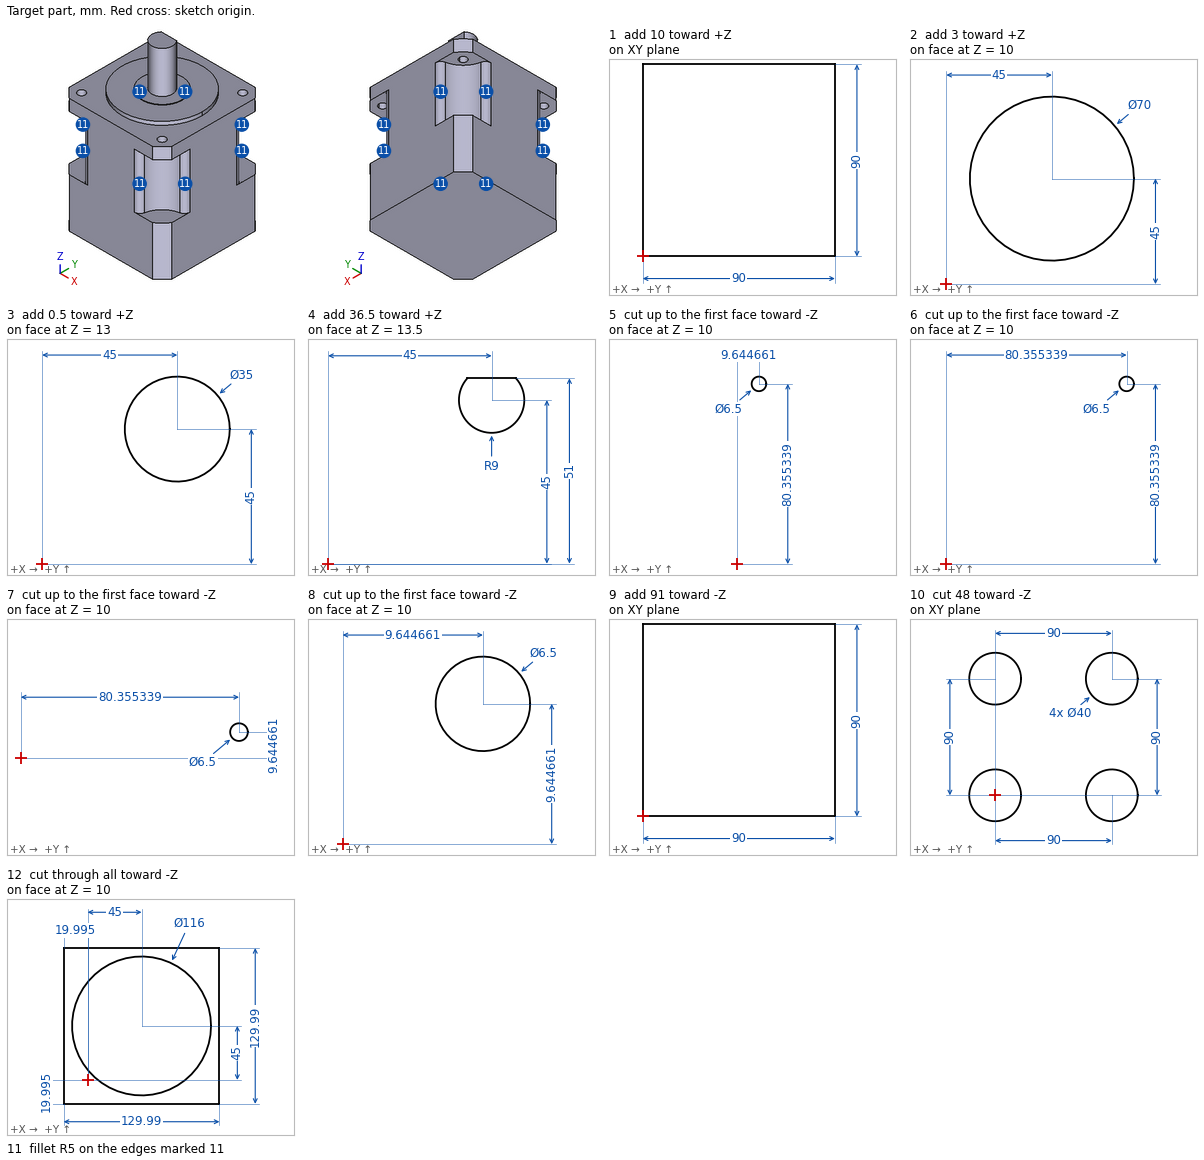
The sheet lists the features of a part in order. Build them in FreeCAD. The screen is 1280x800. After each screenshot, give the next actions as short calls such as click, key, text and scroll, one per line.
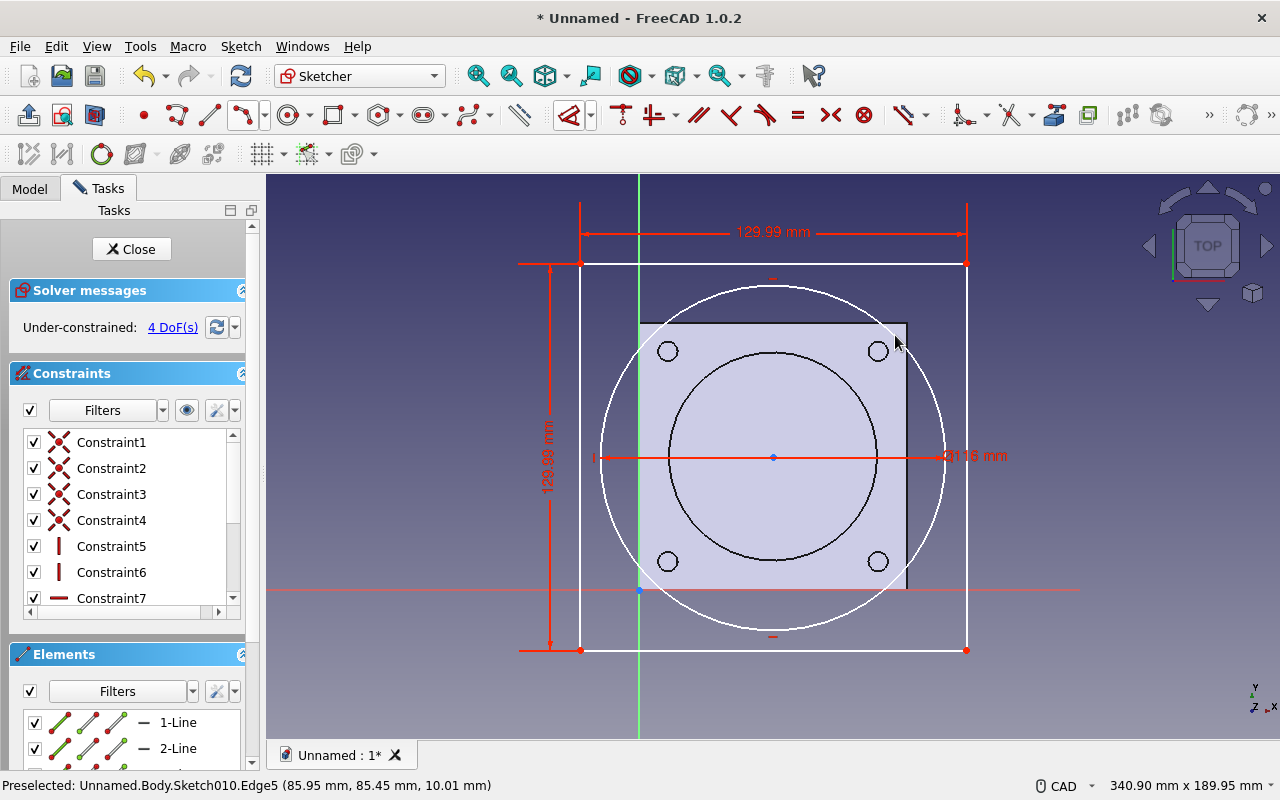
click(773, 458)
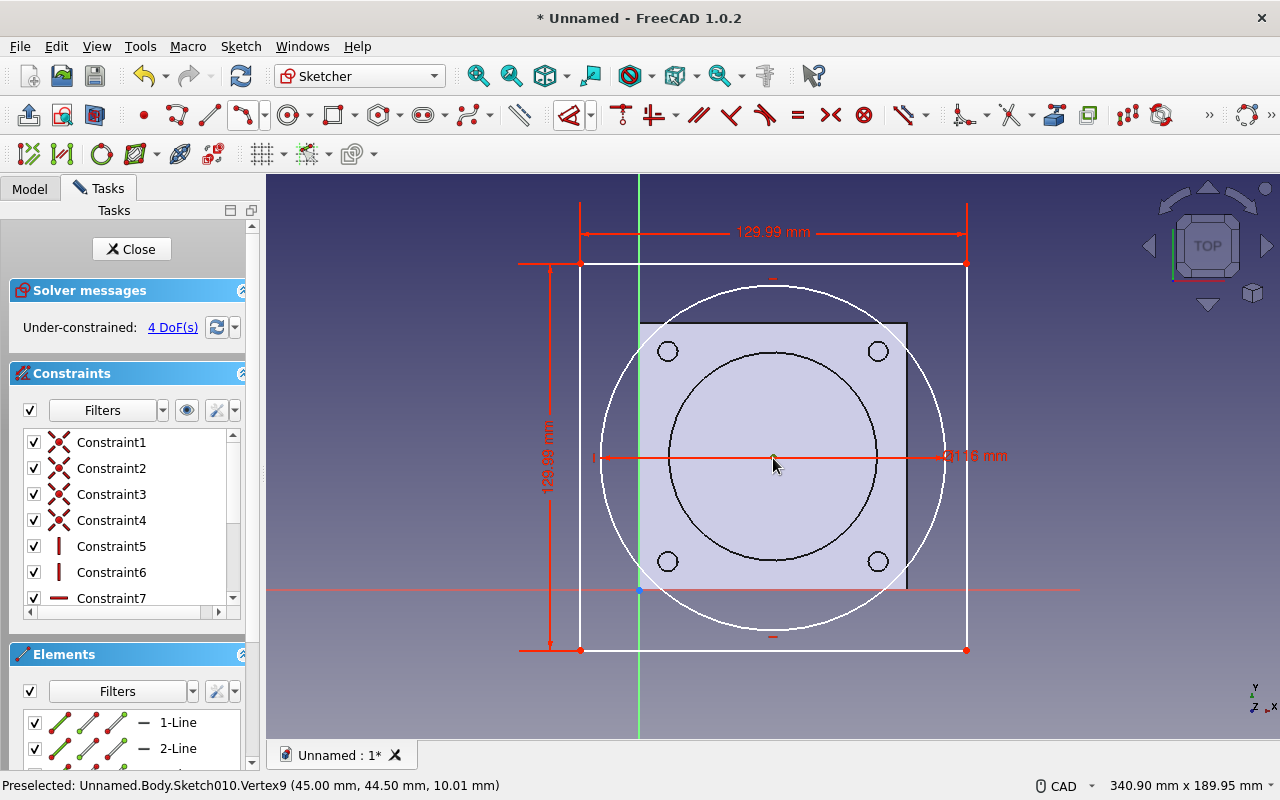
key(l)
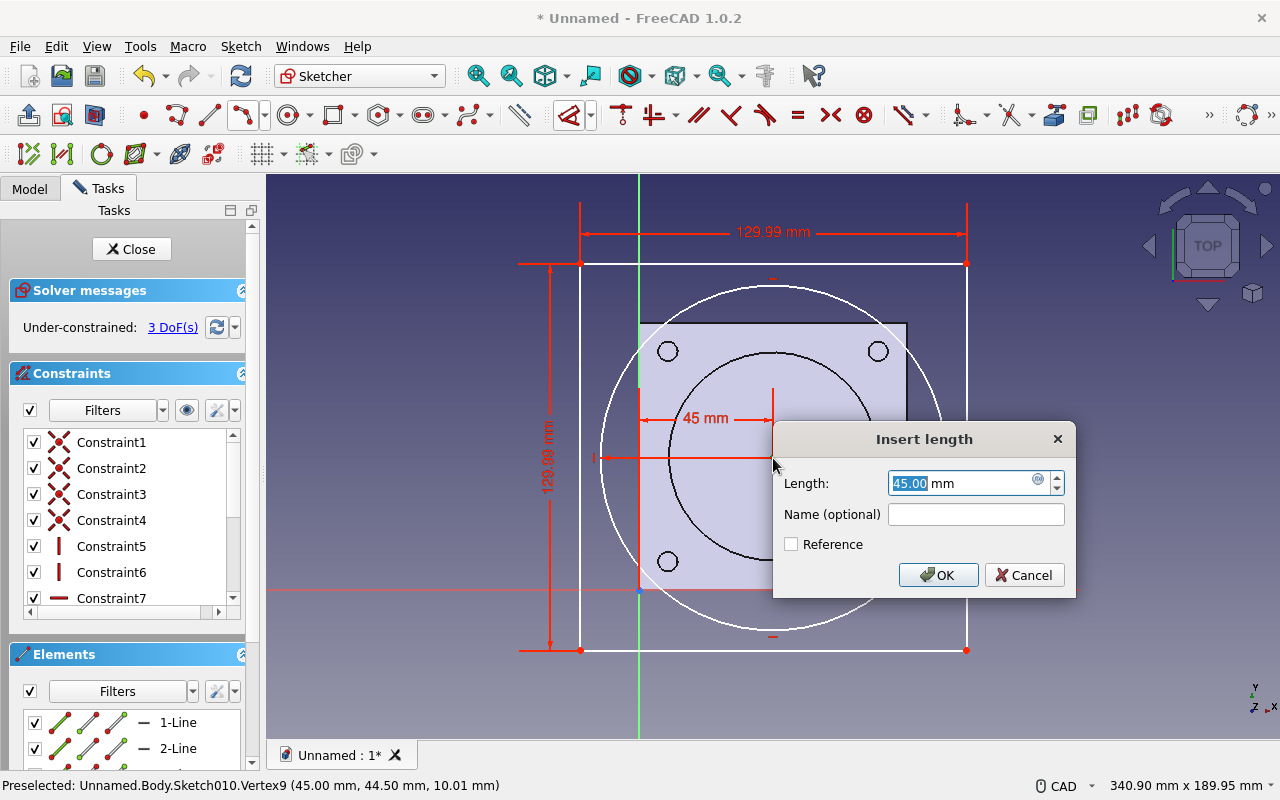
text(45)
key(Return)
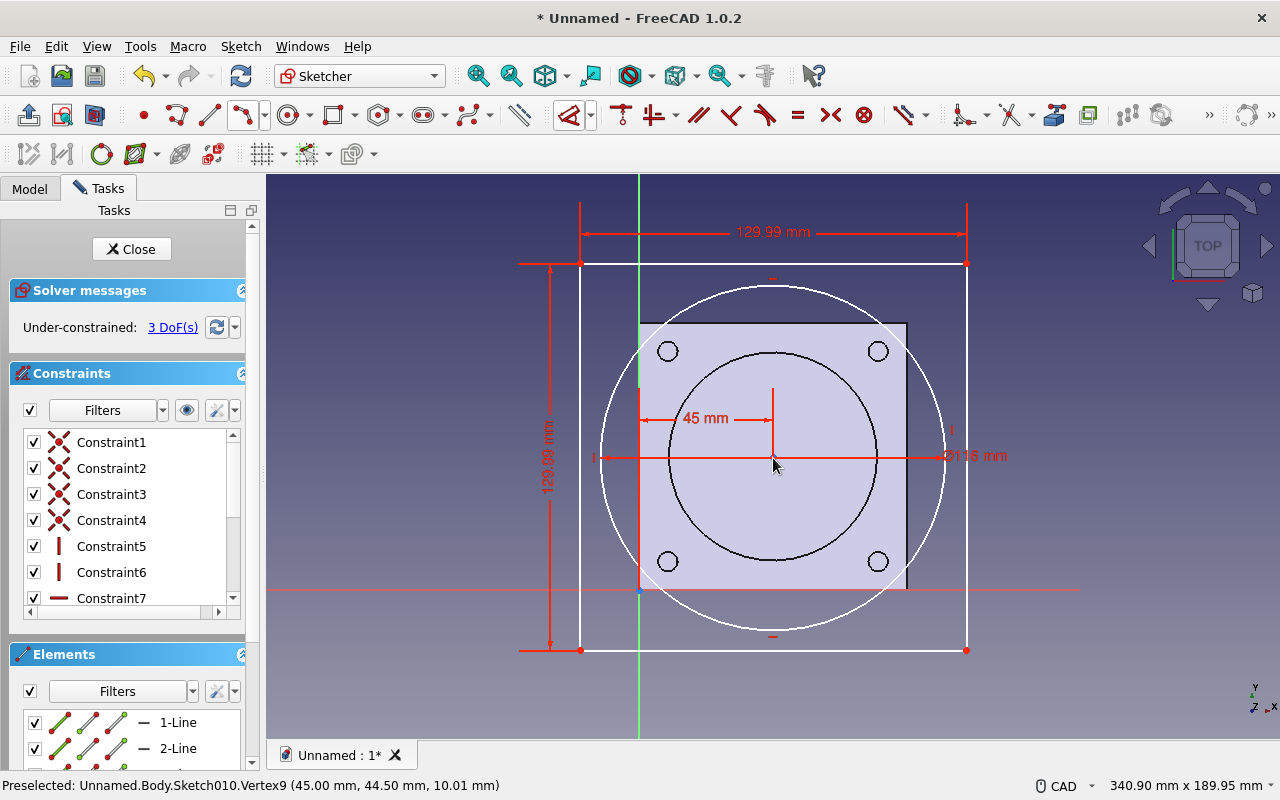
click(773, 458)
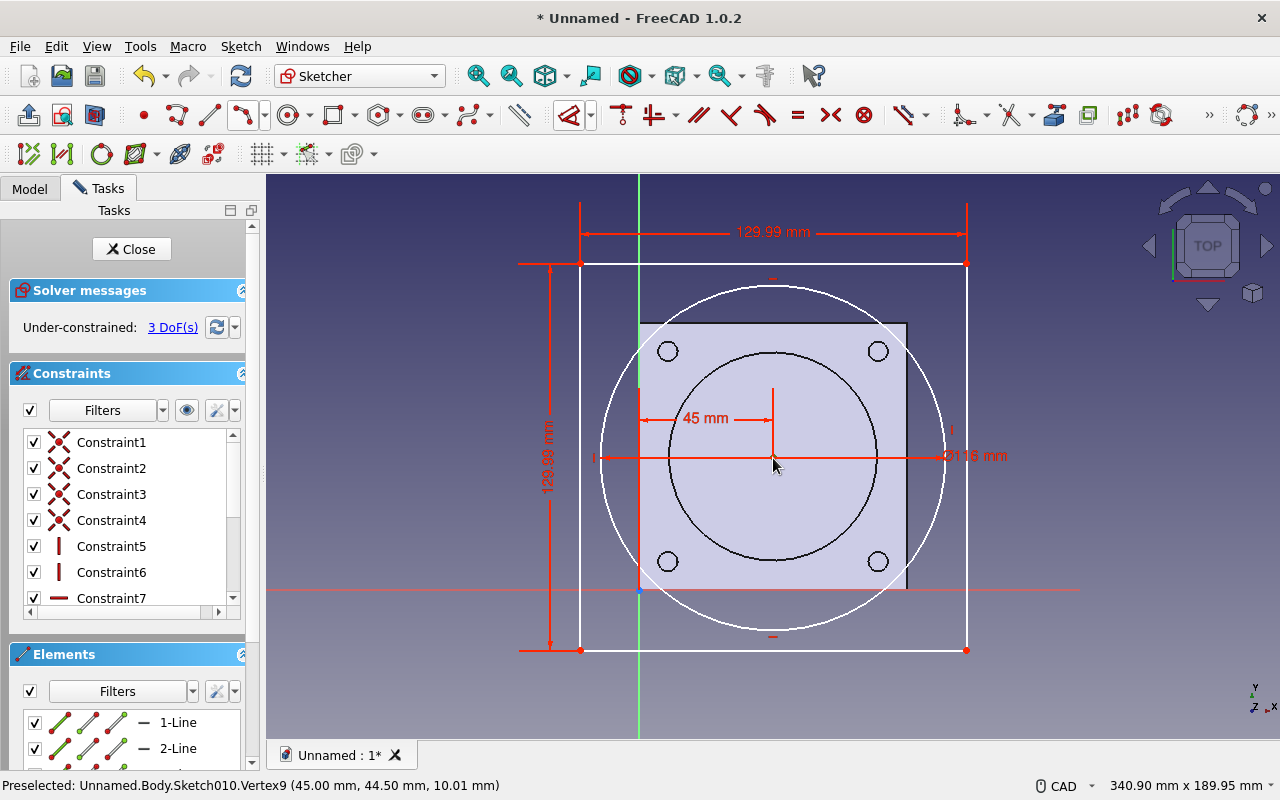
key(i)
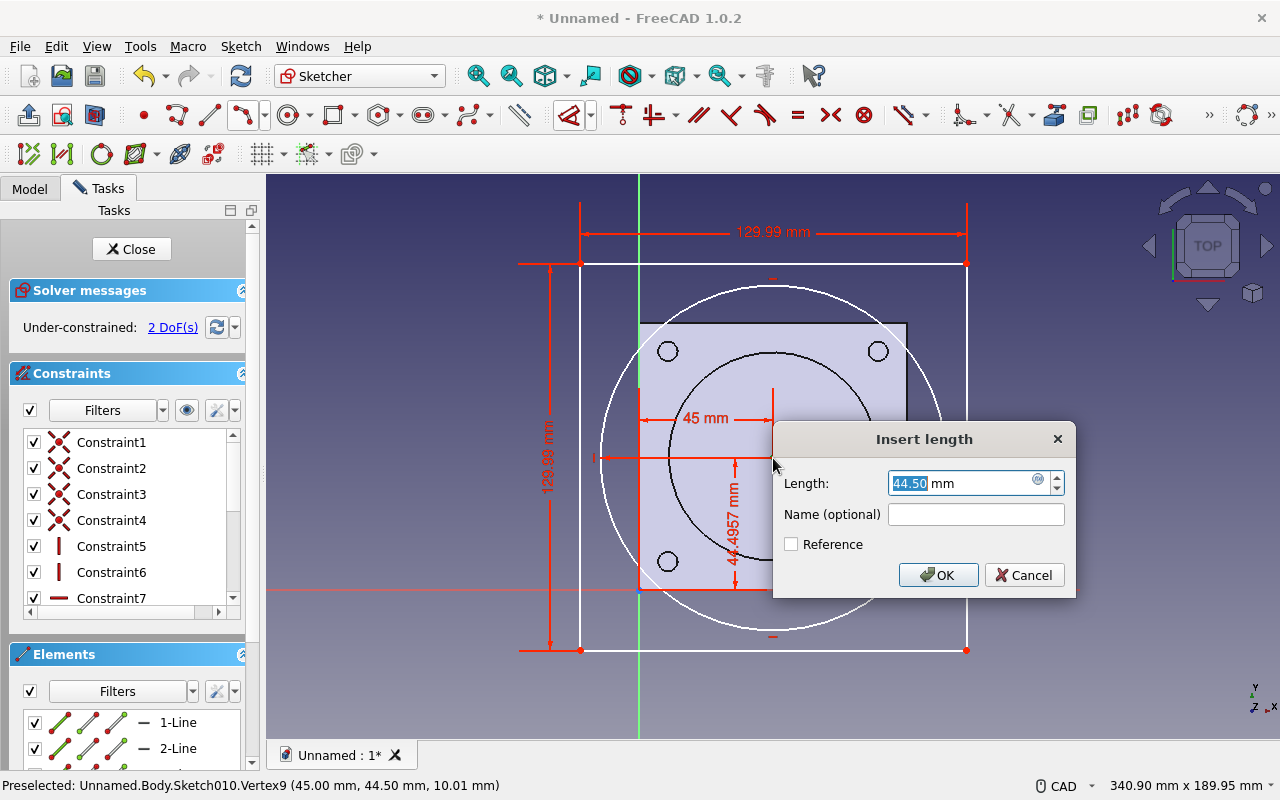
text(45)
key(Return)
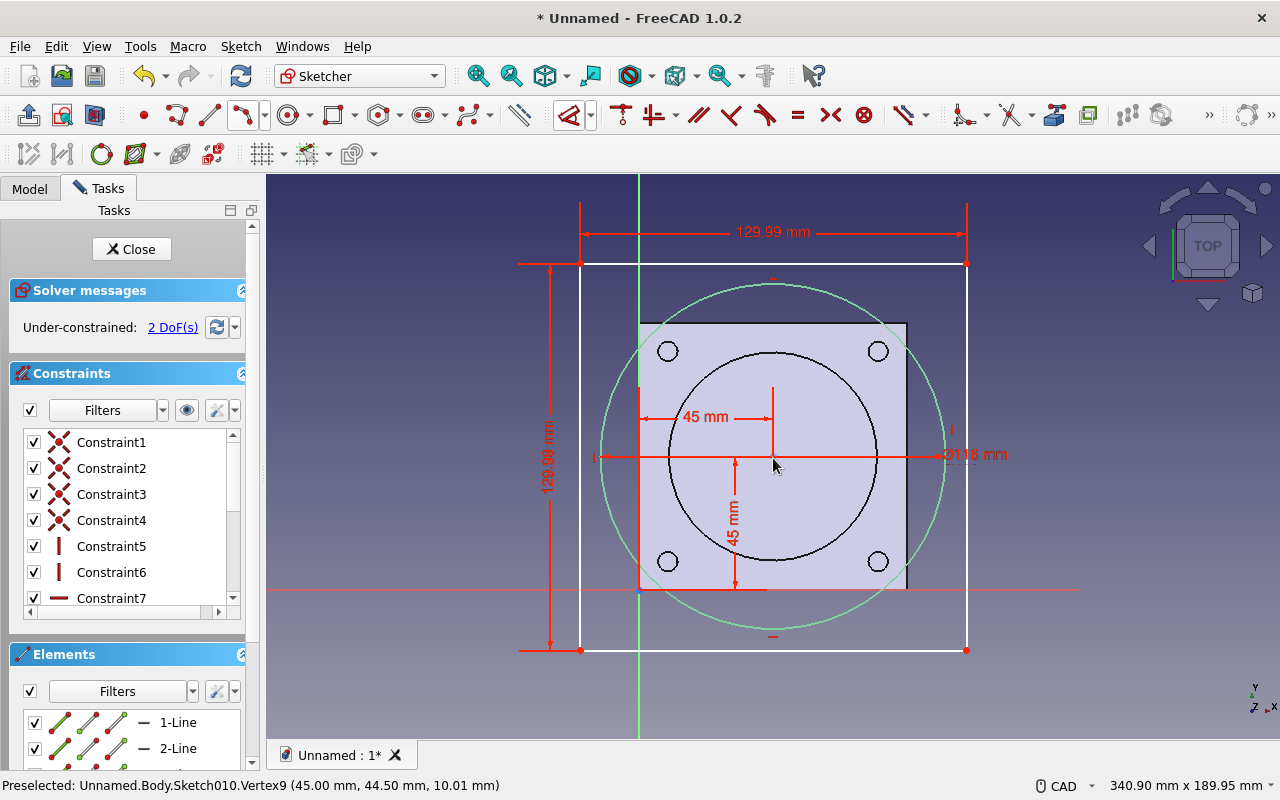
click(580, 264)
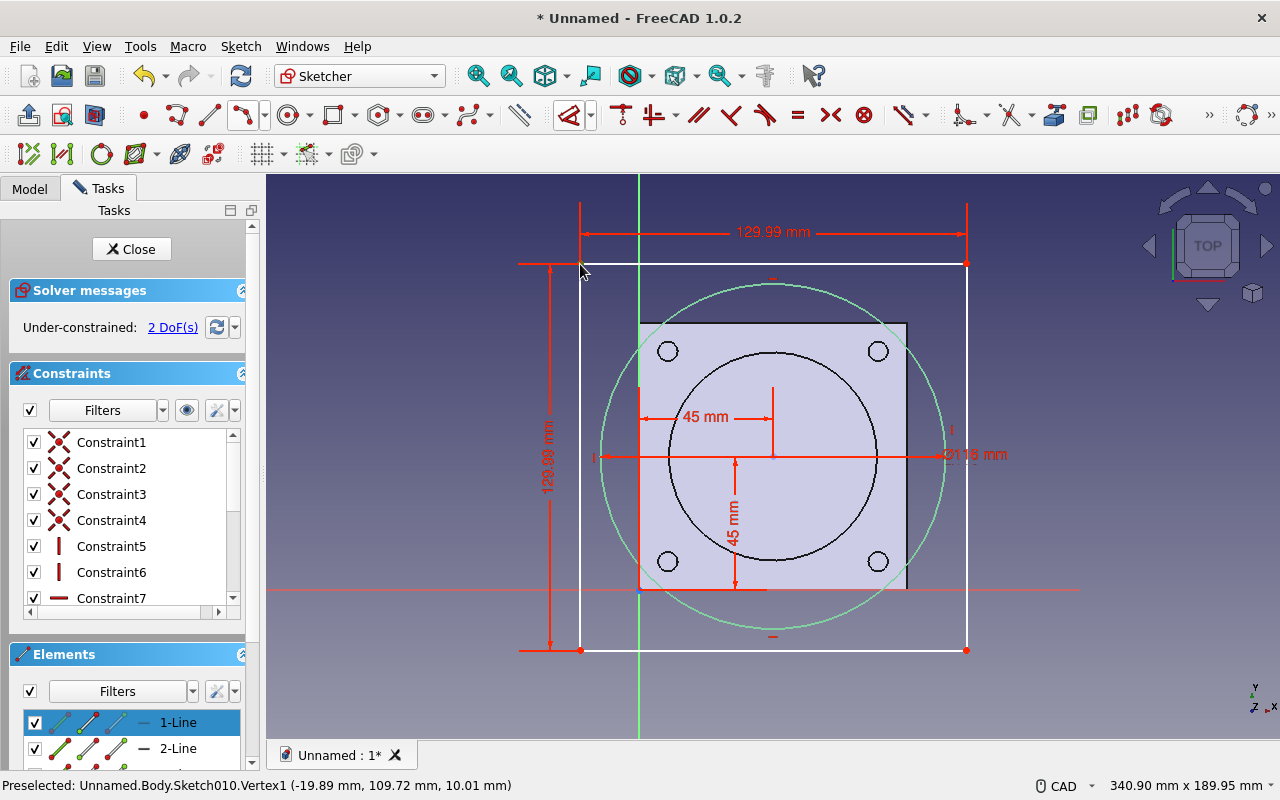
key(l)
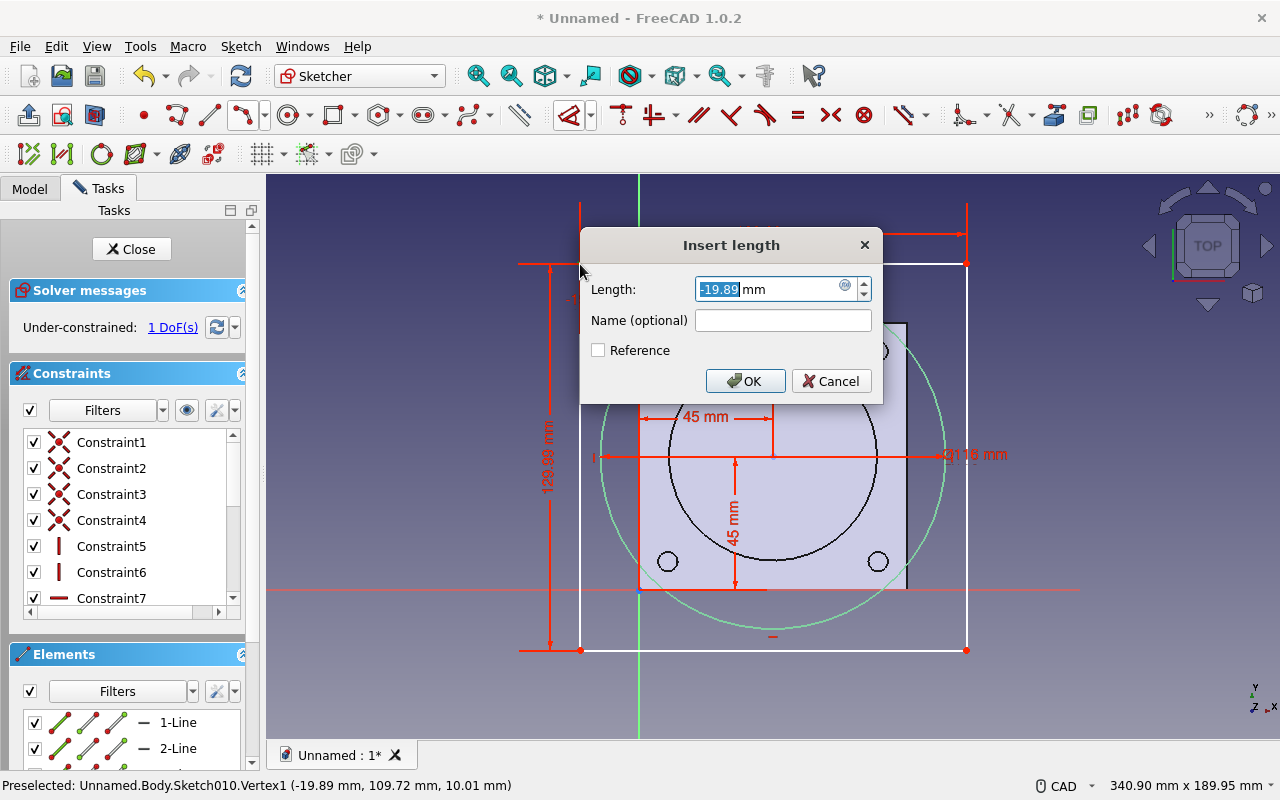
text(-19.995)
key(Return)